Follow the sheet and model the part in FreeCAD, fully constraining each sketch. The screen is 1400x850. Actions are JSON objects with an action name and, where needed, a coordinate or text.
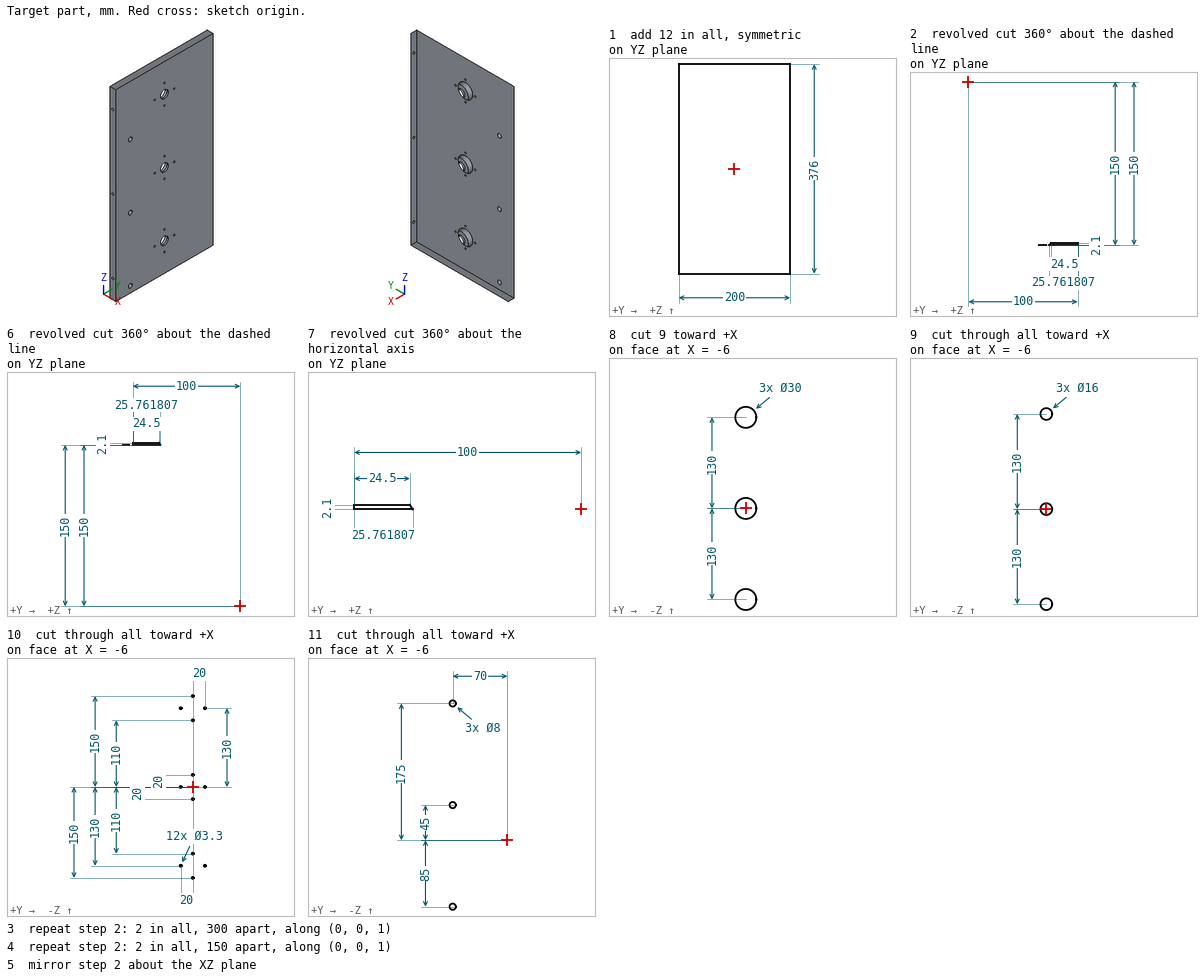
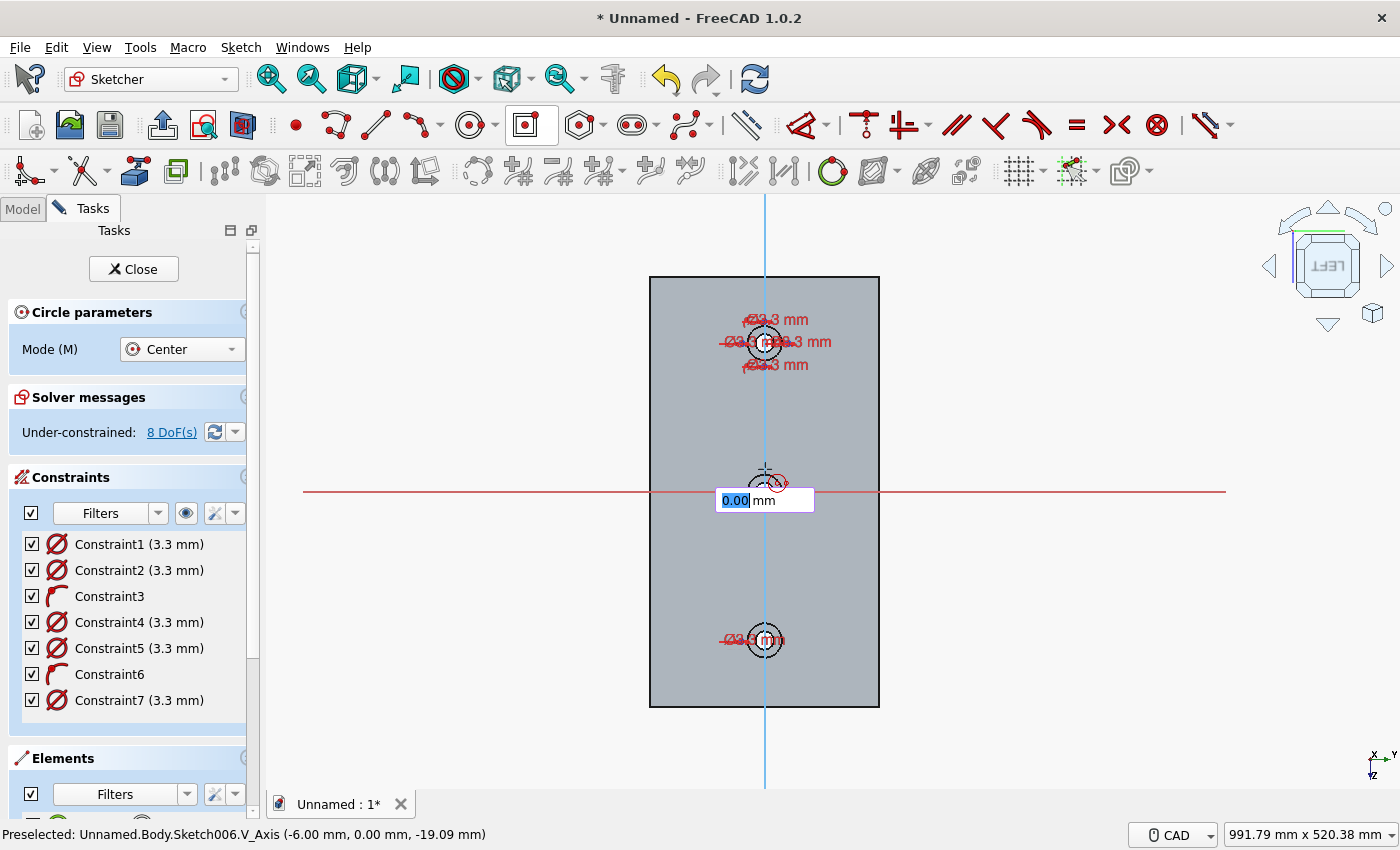
{"action": "scroll", "coordinate": [767, 468], "scroll_direction": "up", "scroll_amount": 11}
{"action": "mouse_move", "coordinate": [759, 467]}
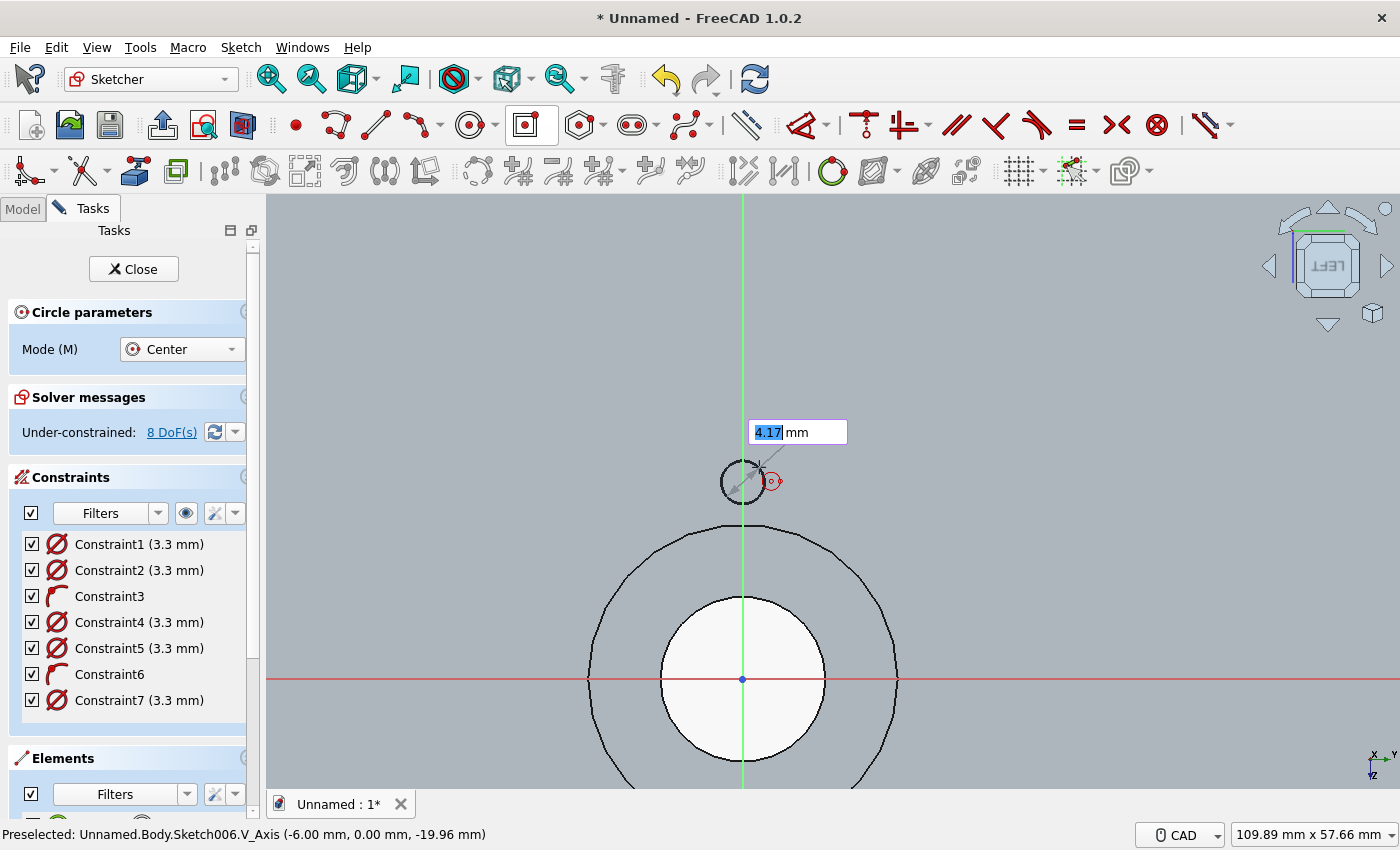
{"action": "type", "text": "3.3"}
{"action": "key", "text": "Return"}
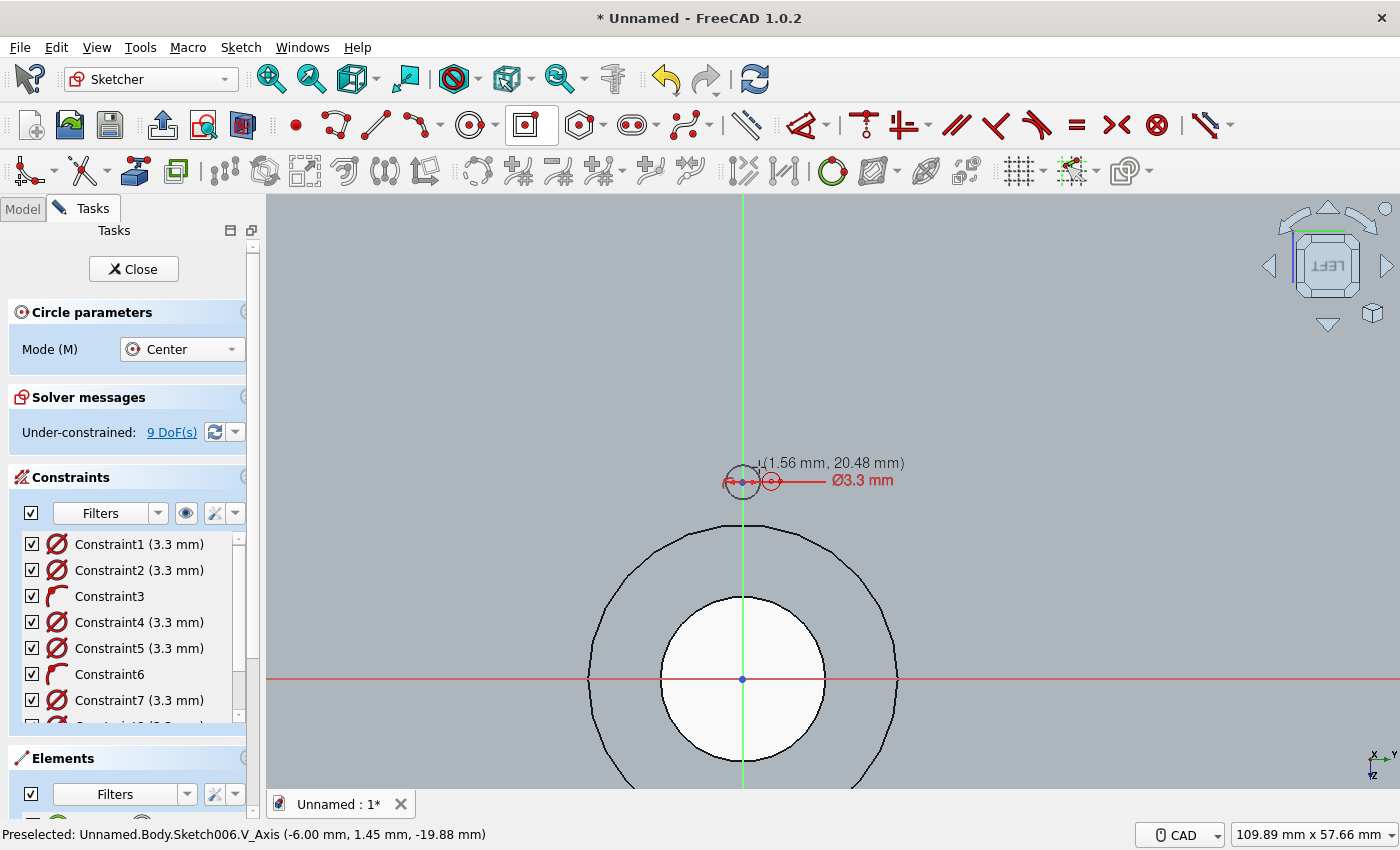
{"action": "scroll", "coordinate": [949, 679], "scroll_direction": "up", "scroll_amount": 2}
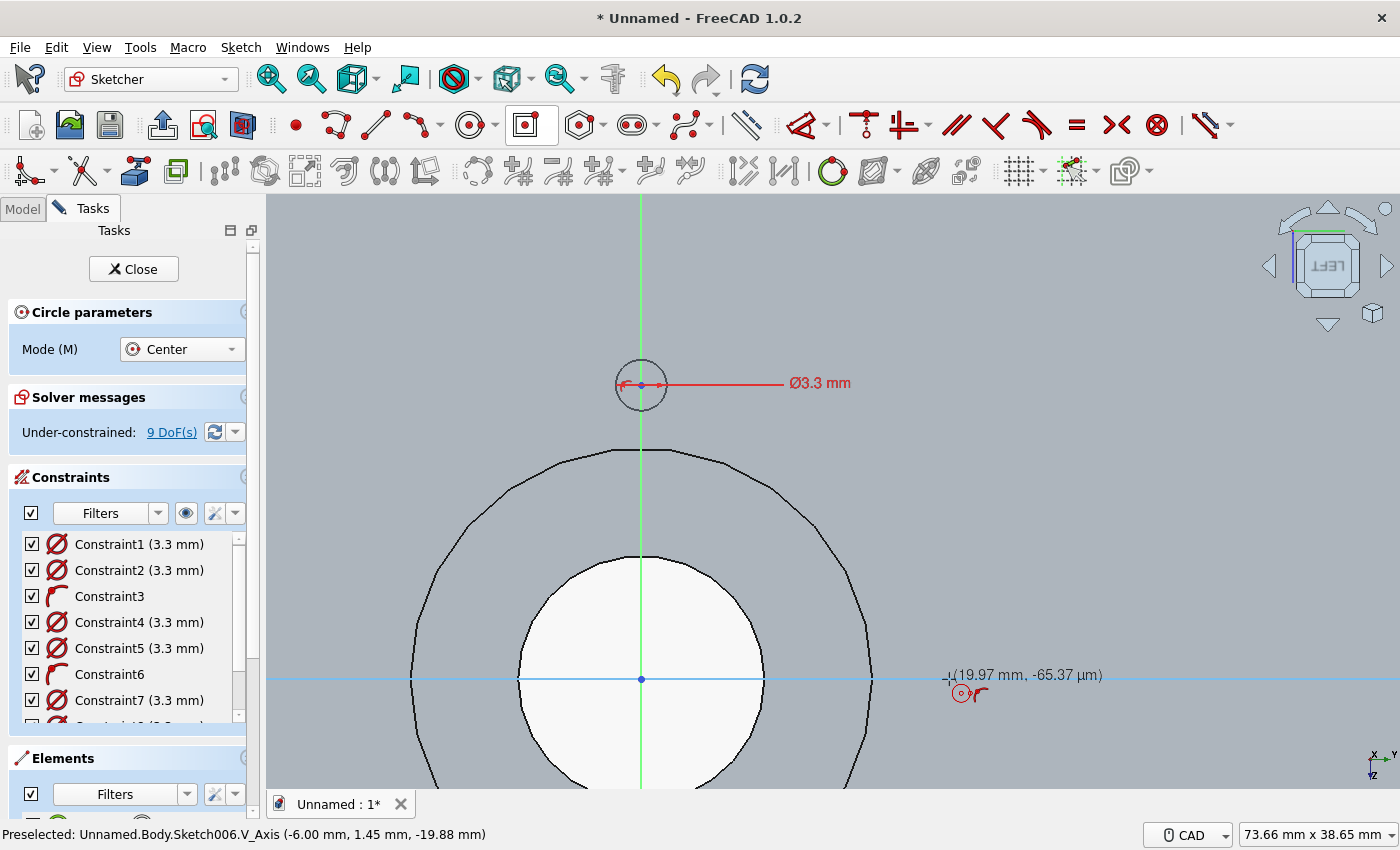
{"action": "scroll", "coordinate": [774, 476], "scroll_direction": "down", "scroll_amount": 13}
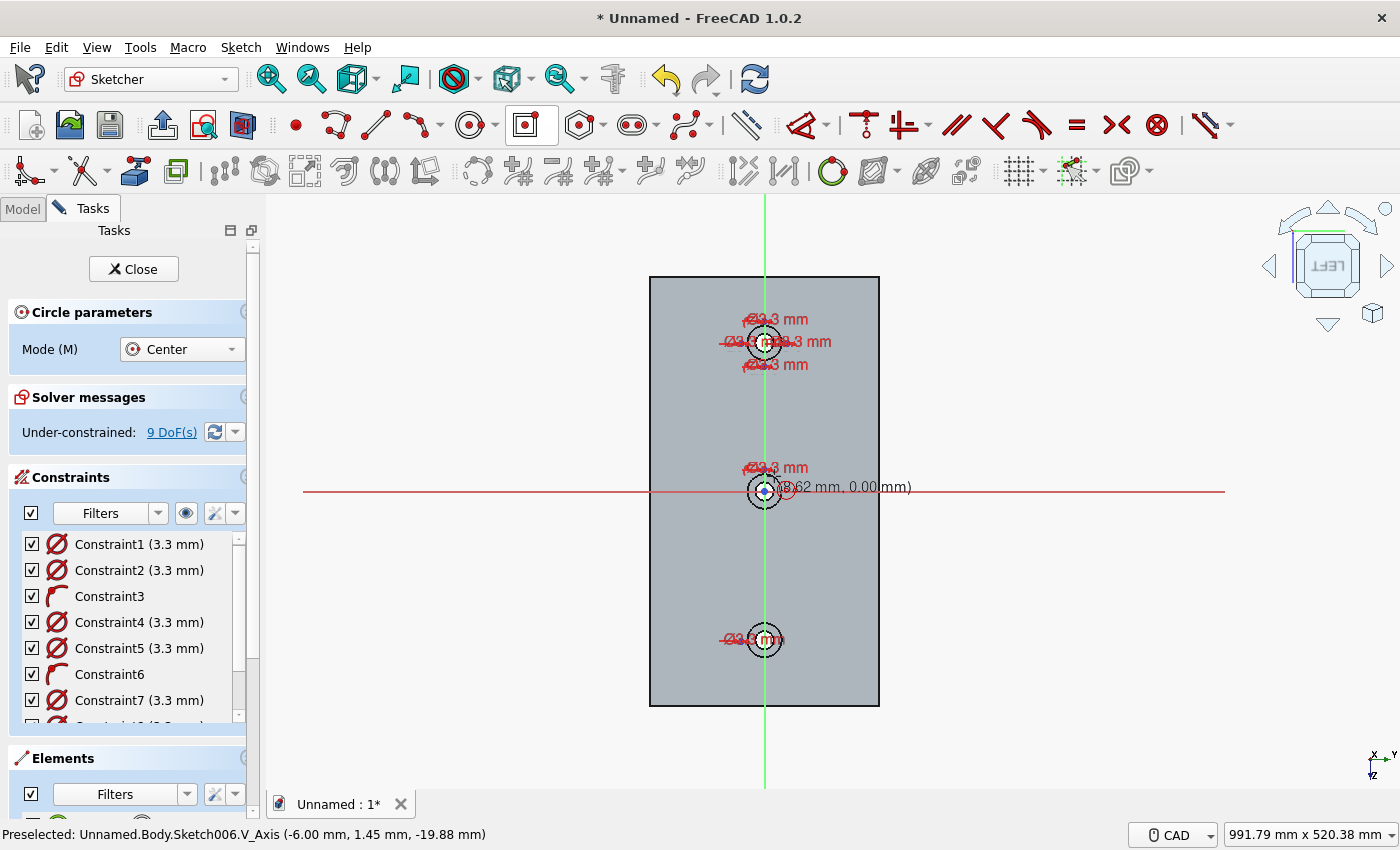
{"action": "left_click", "coordinate": [787, 492]}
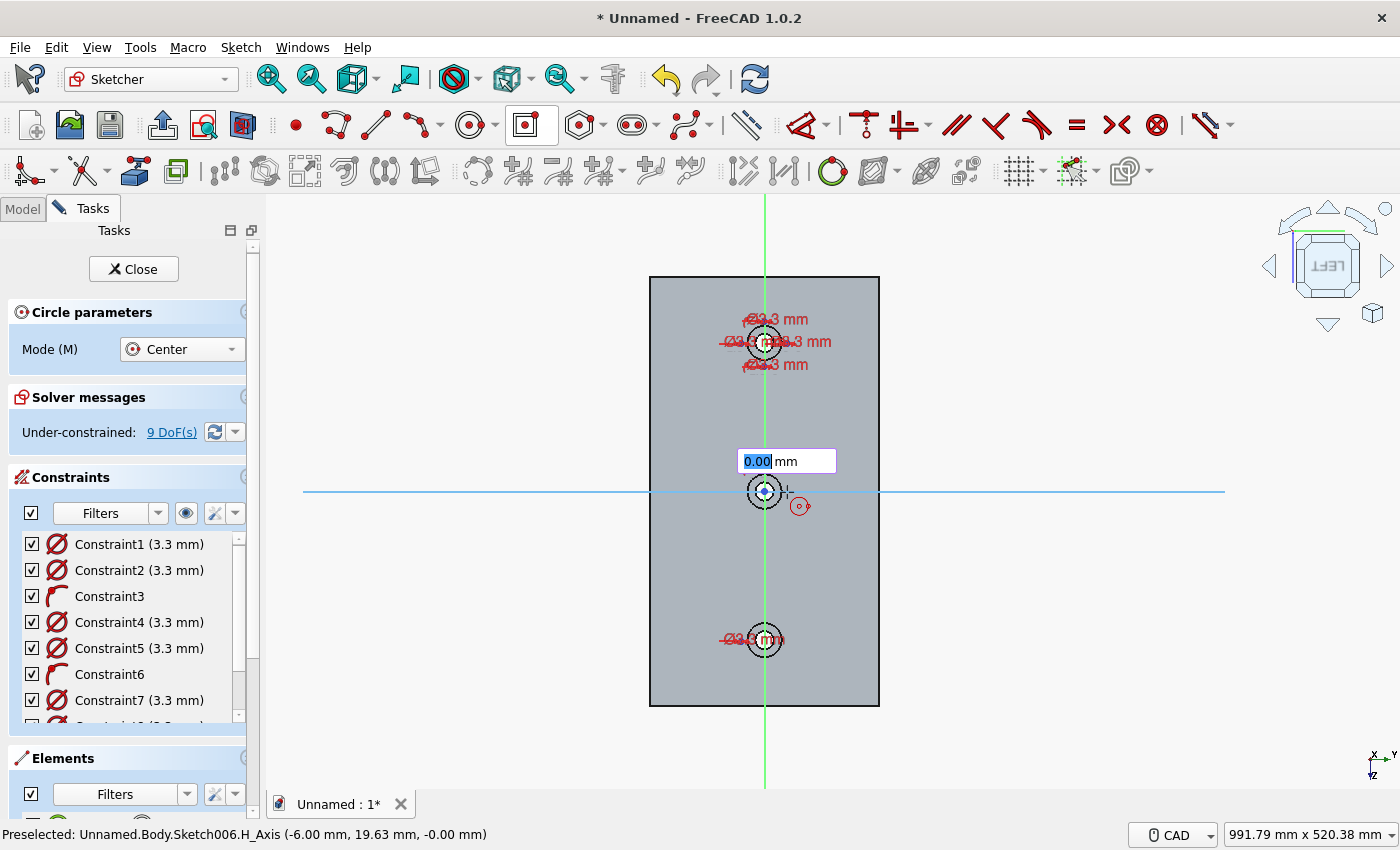
{"action": "scroll", "coordinate": [787, 493], "scroll_direction": "up", "scroll_amount": 11}
{"action": "mouse_move", "coordinate": [781, 492]}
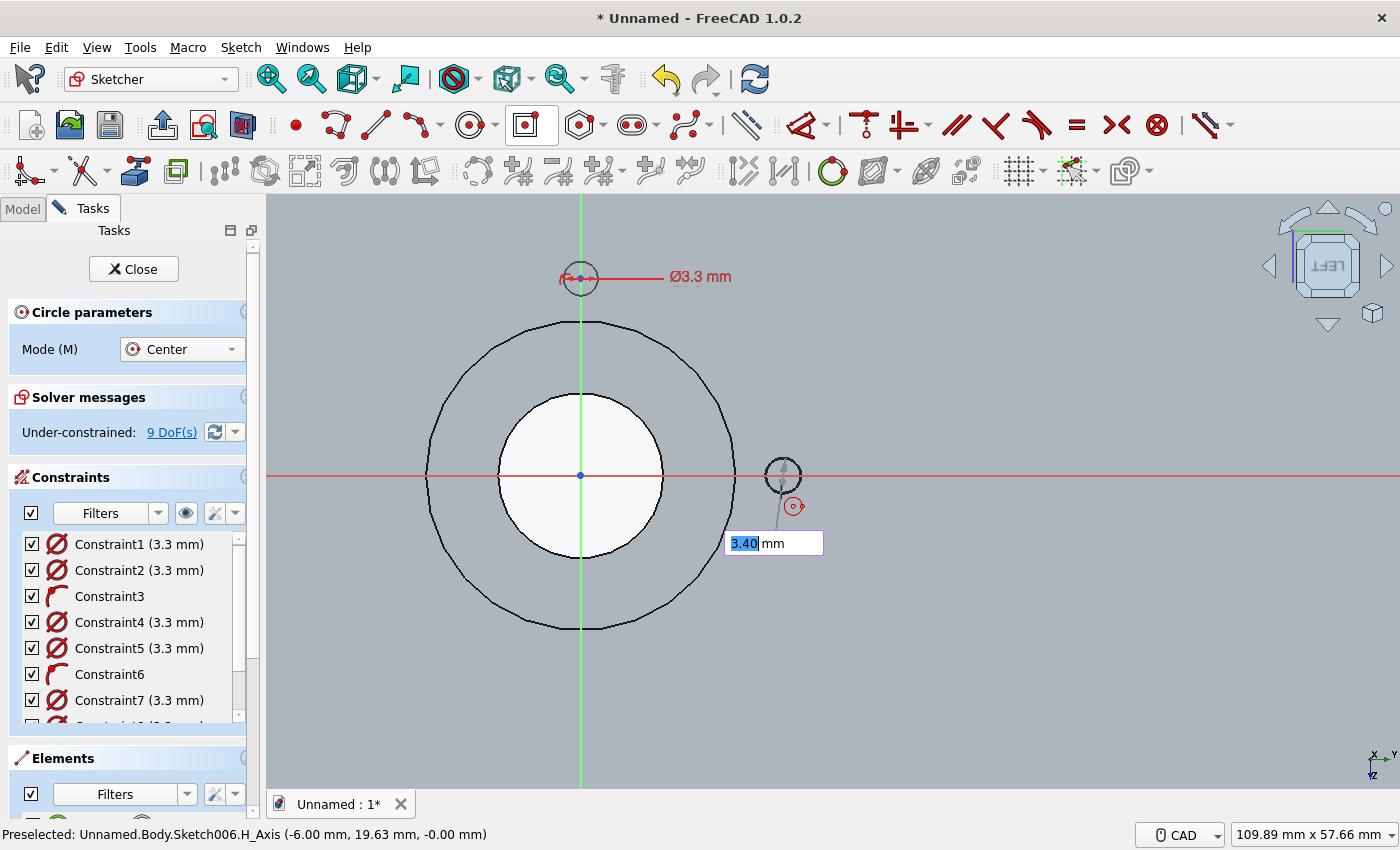
{"action": "type", "text": "3.3"}
{"action": "key", "text": "Return"}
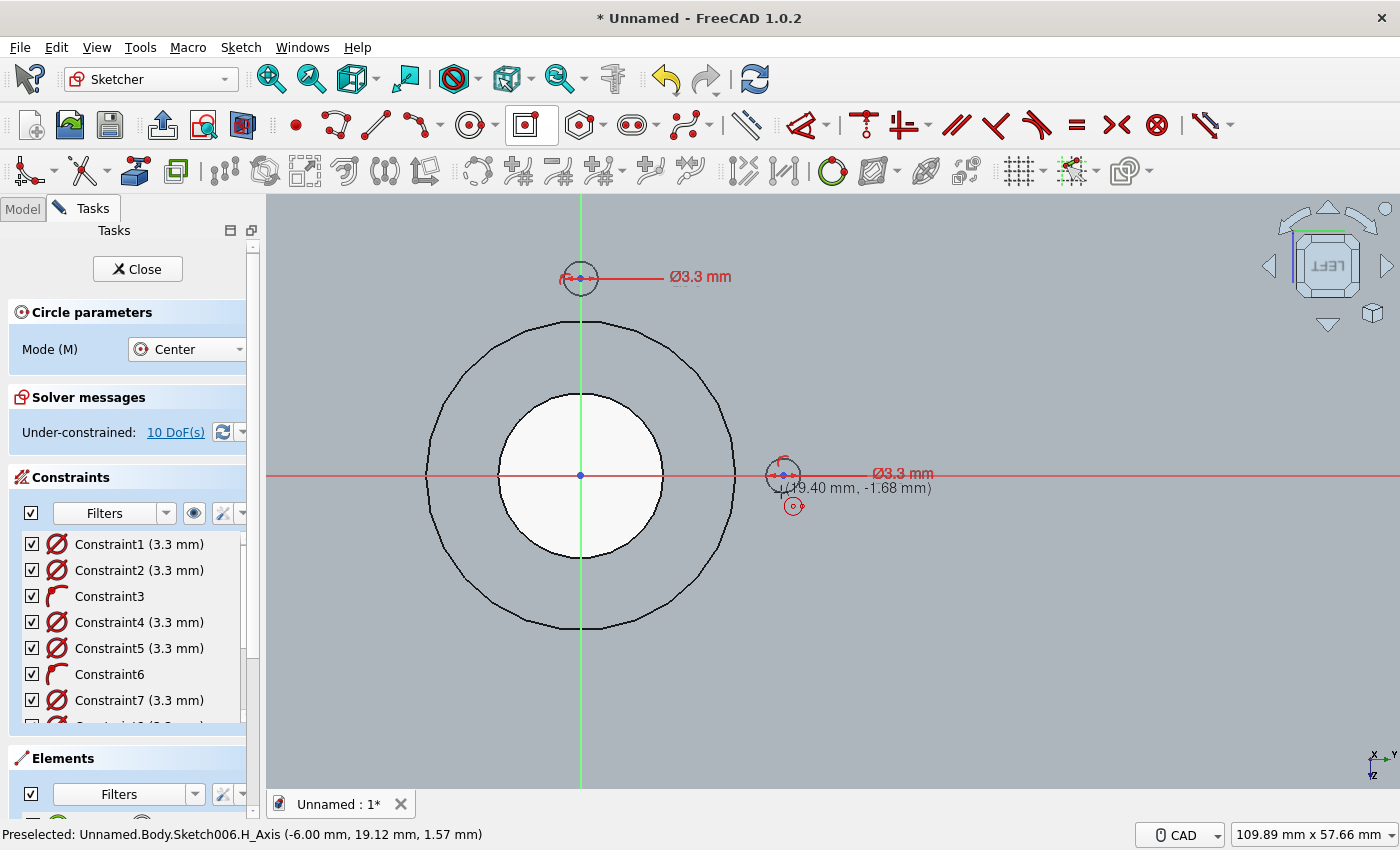
{"action": "scroll", "coordinate": [581, 682], "scroll_direction": "up", "scroll_amount": 2}